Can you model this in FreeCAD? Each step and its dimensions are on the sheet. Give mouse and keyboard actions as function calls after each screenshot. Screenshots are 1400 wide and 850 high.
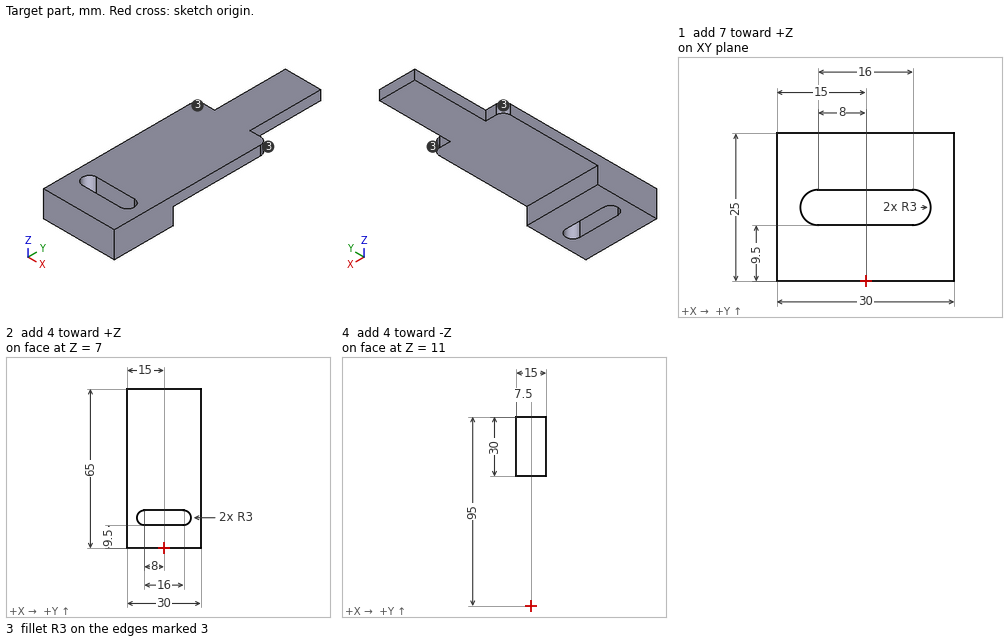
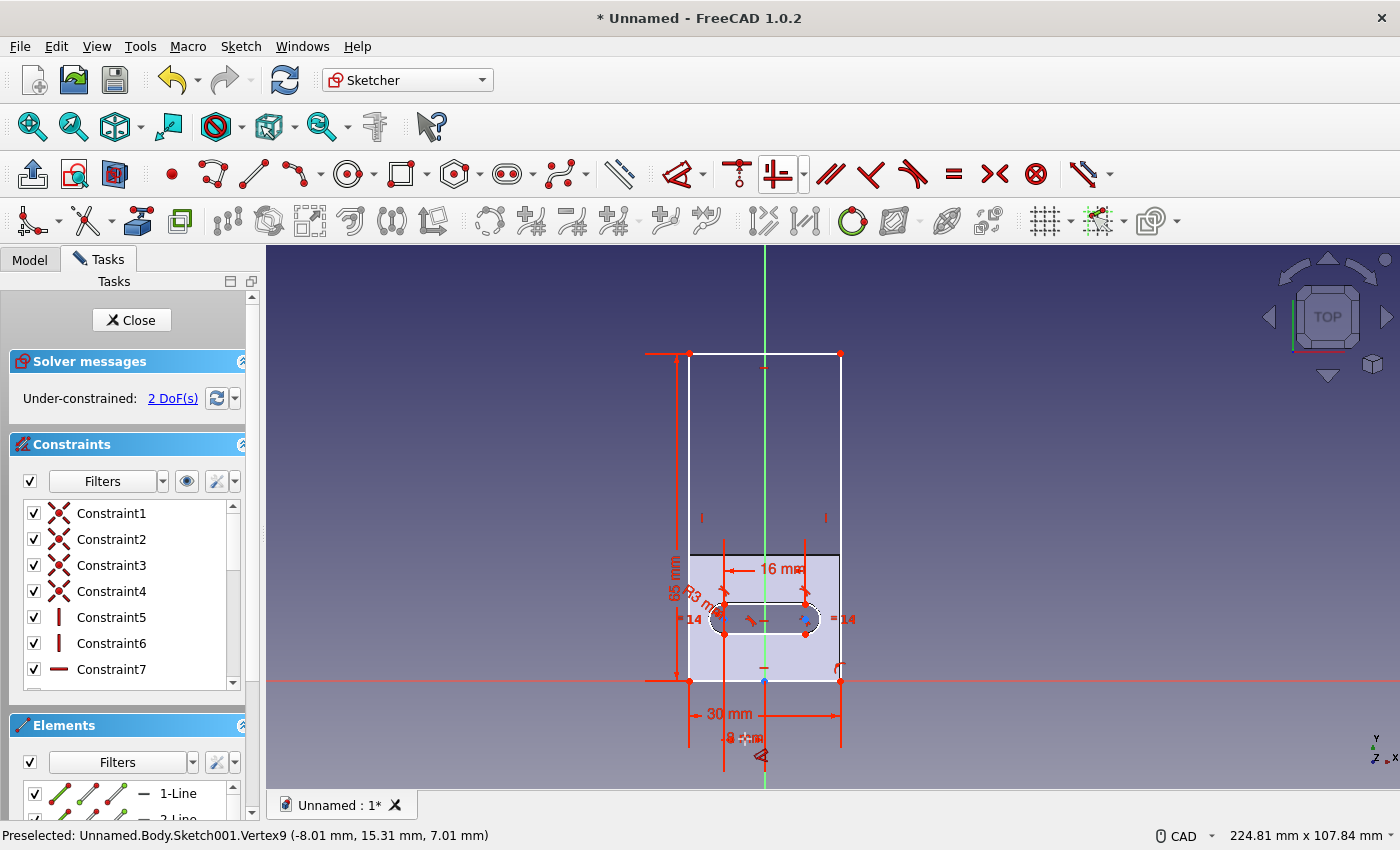
click(689, 354)
click(727, 320)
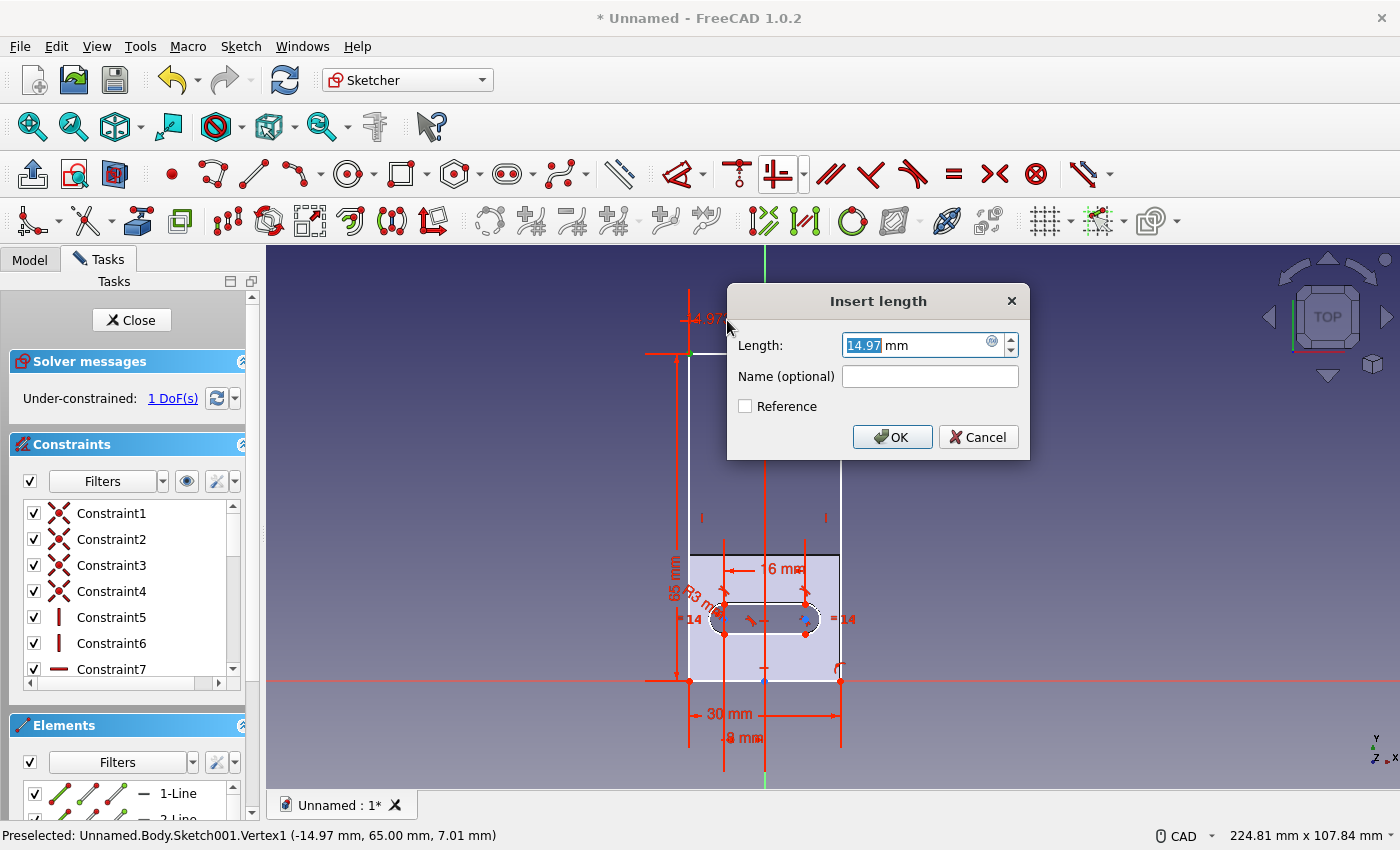
text(15)
key(Return)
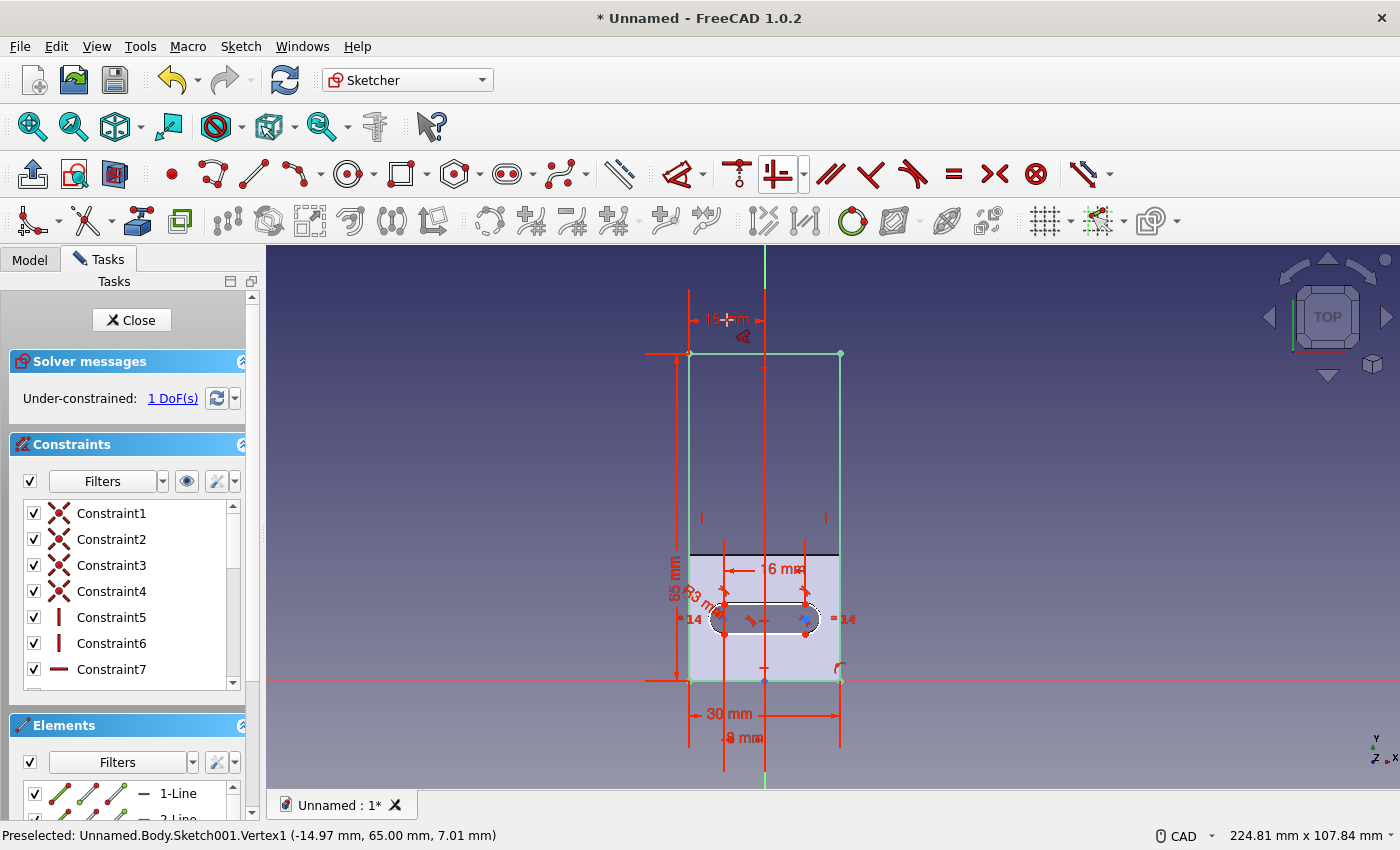
click(724, 634)
click(799, 658)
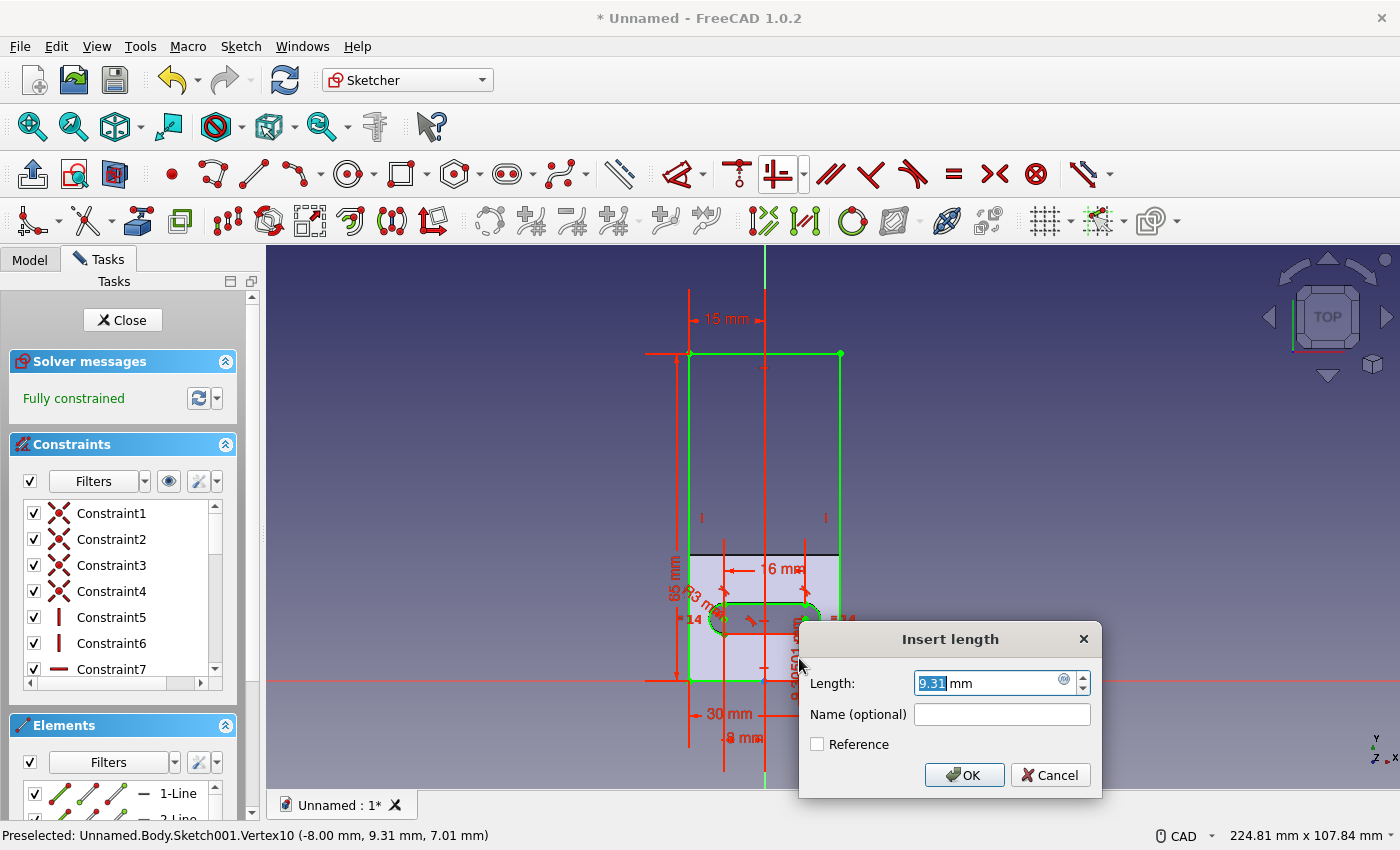
text(9.5)
key(Return)
key(Escape)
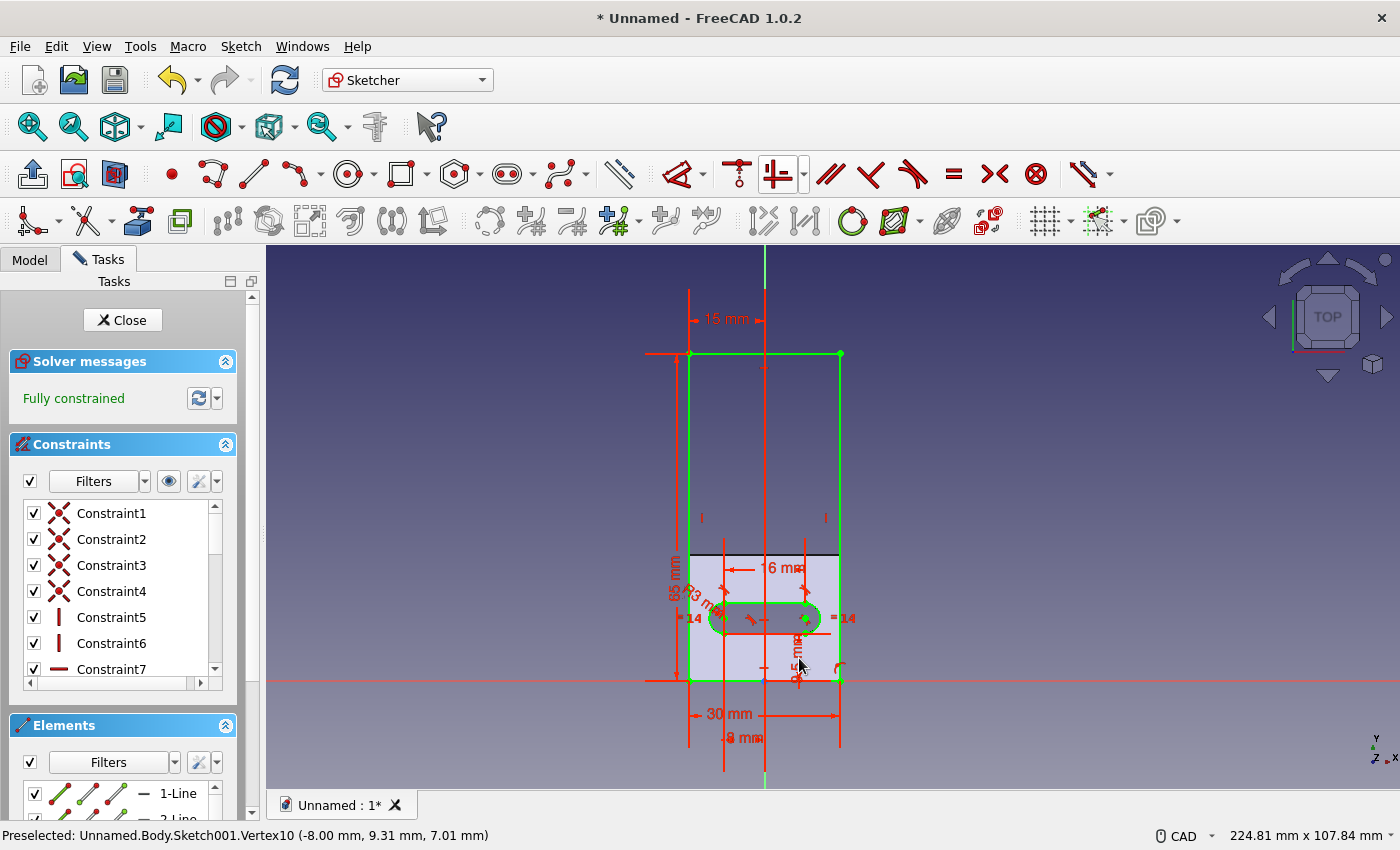
click(123, 320)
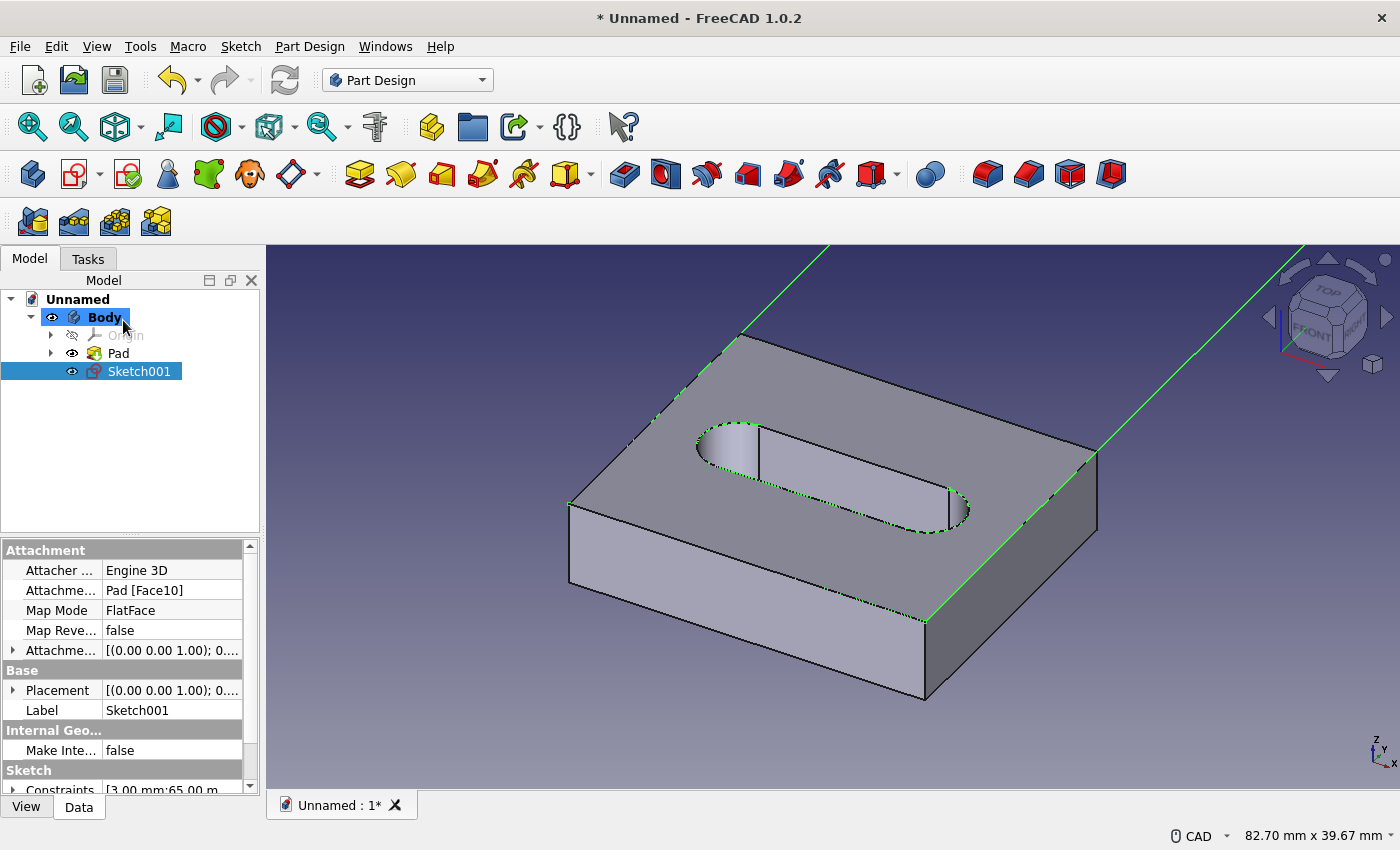
click(360, 174)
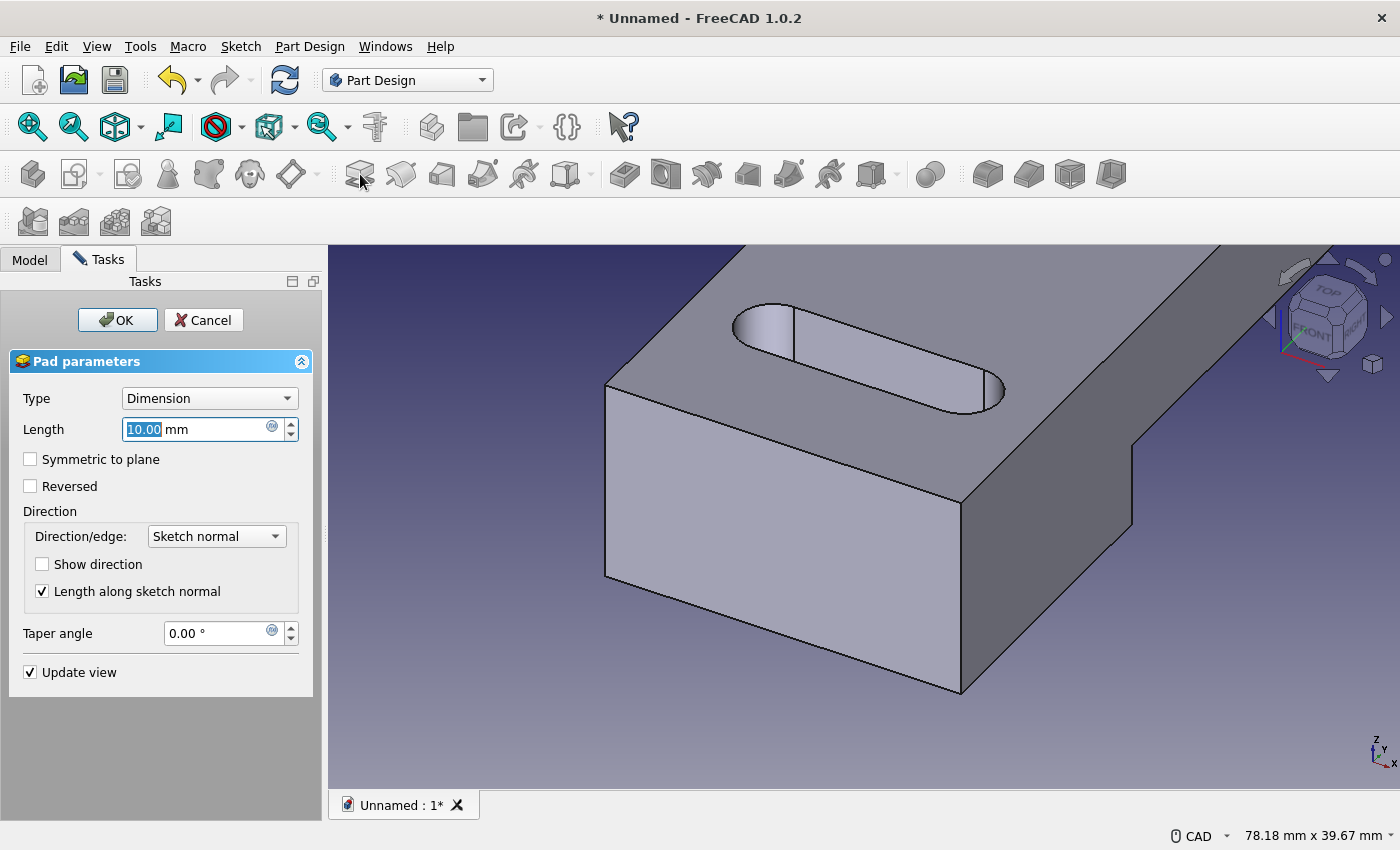
text(4)
key(Tab)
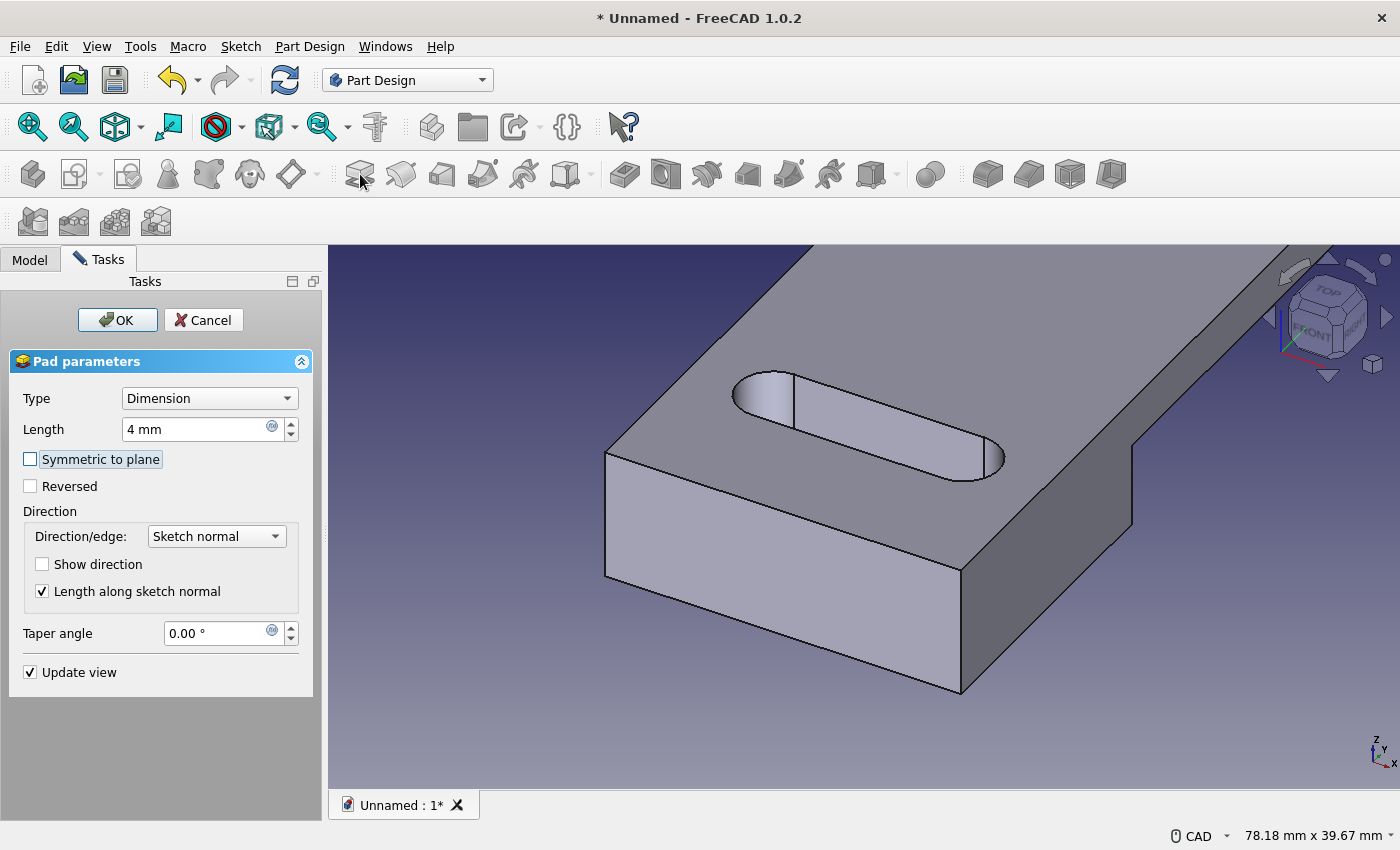
click(118, 320)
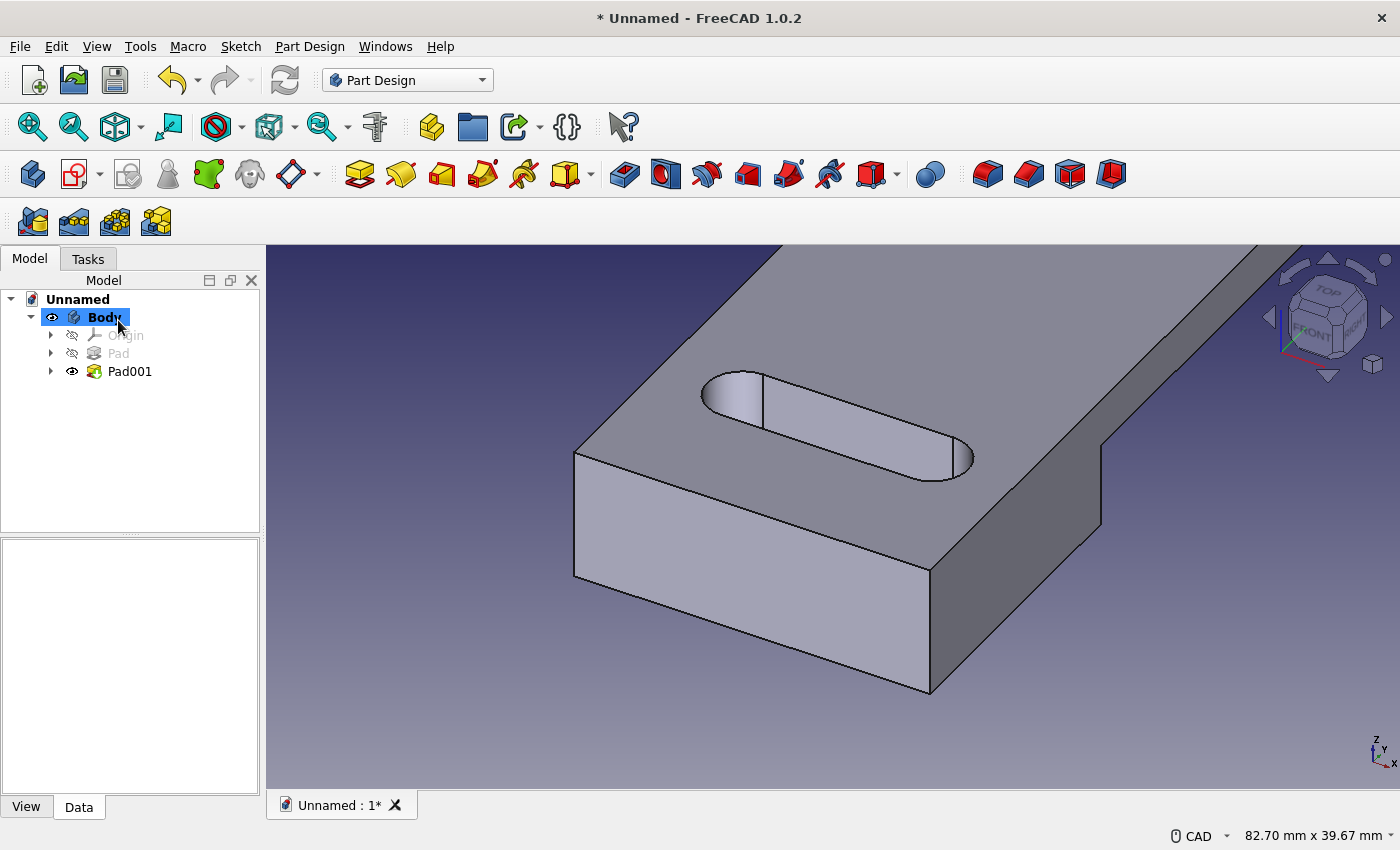
click(33, 128)